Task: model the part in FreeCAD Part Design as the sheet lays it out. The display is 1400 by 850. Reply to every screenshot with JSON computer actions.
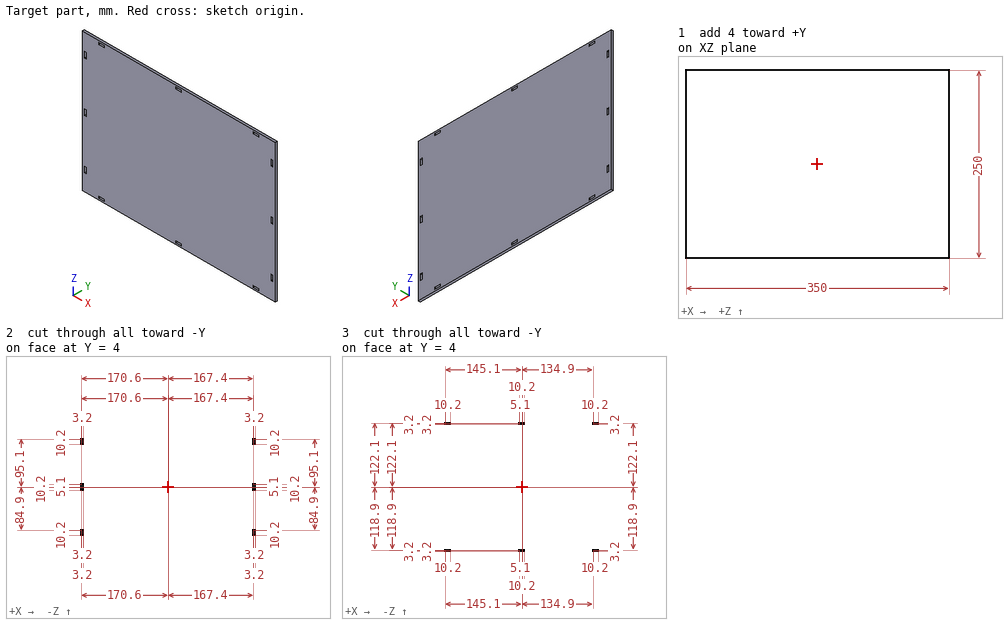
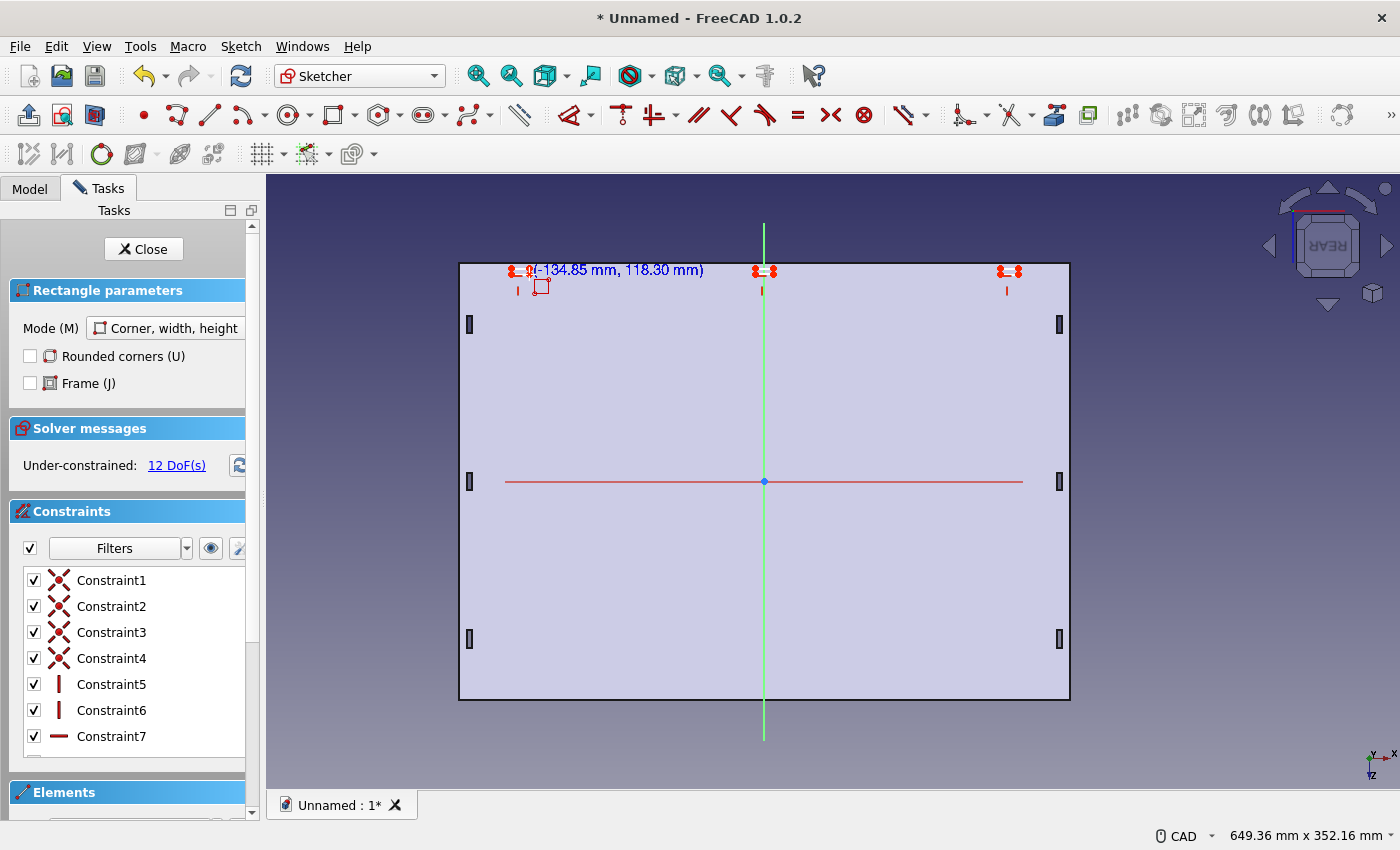
{"action": "scroll", "coordinate": [511, 689], "scroll_direction": "up", "scroll_amount": 6}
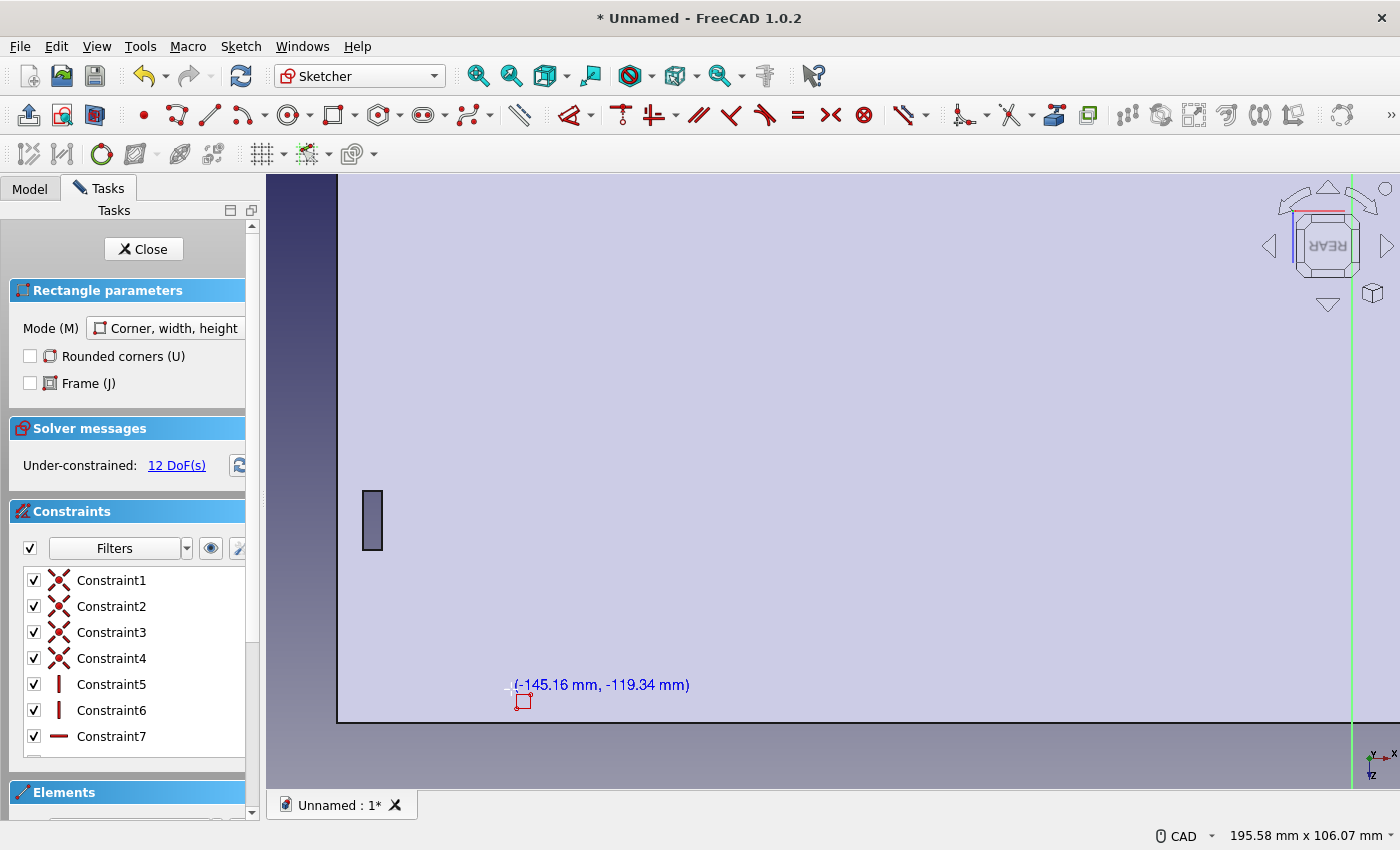
{"action": "scroll", "coordinate": [511, 690], "scroll_direction": "down", "scroll_amount": 6}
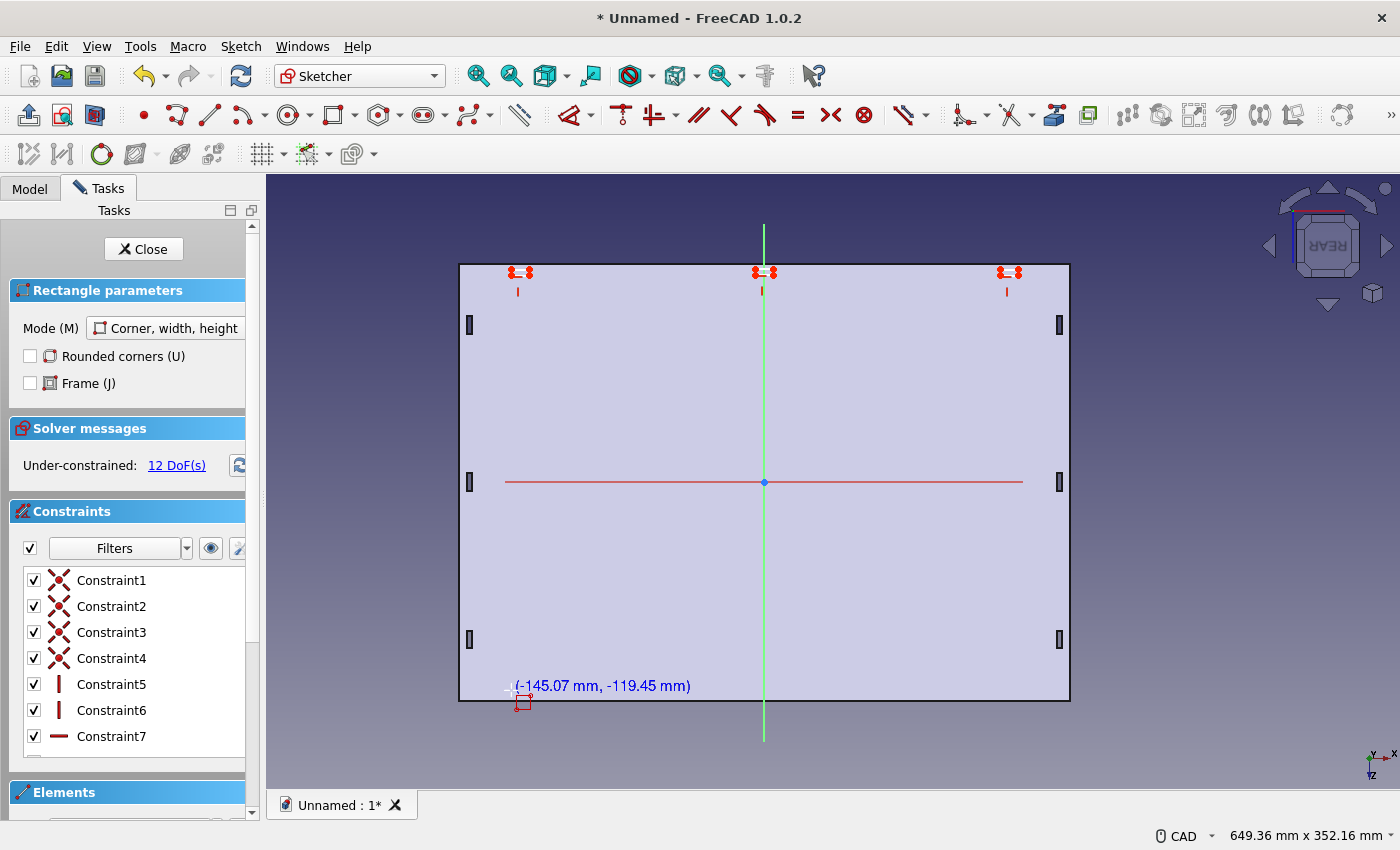
{"action": "left_click", "coordinate": [511, 690]}
{"action": "left_click", "coordinate": [529, 696]}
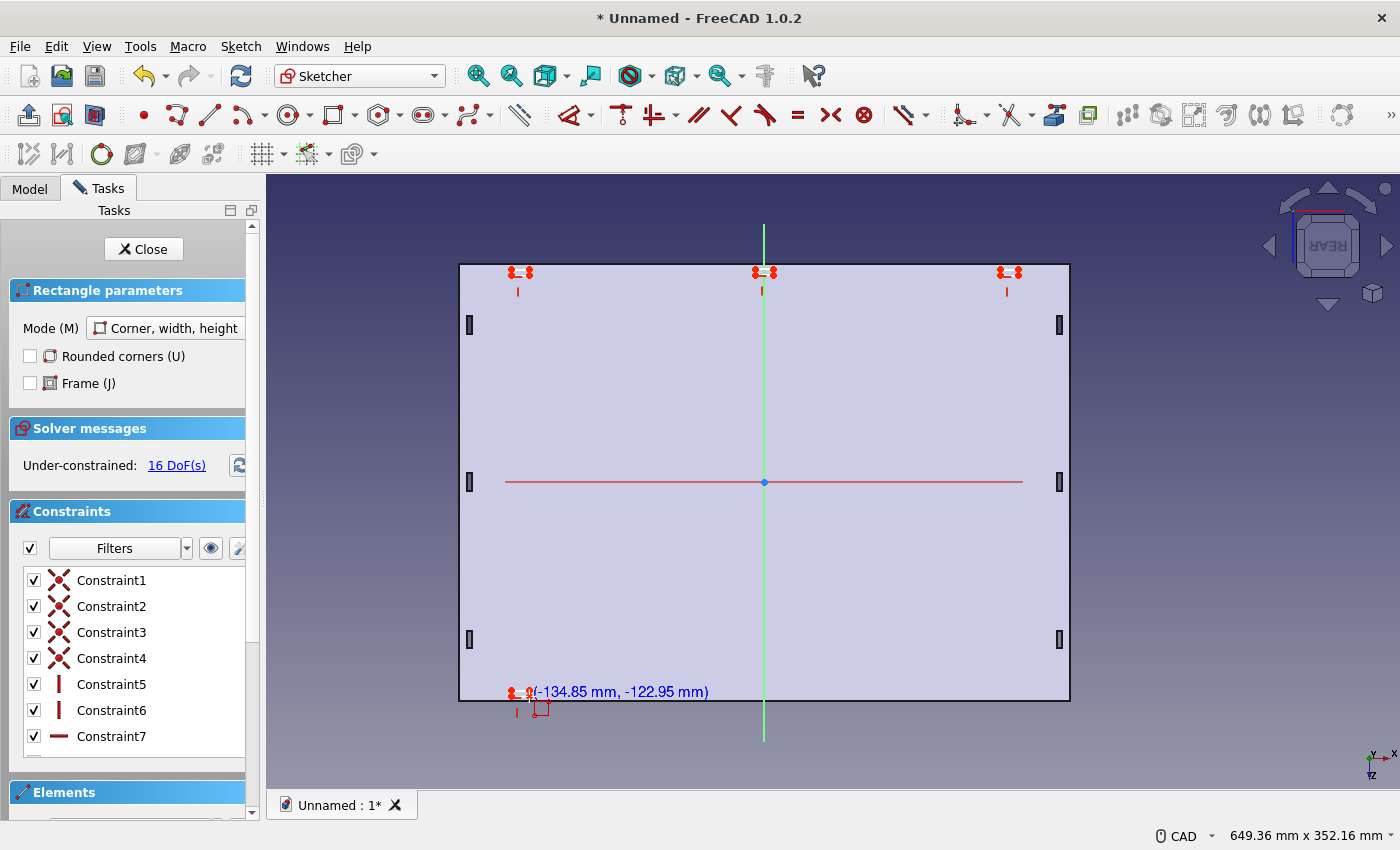
{"action": "scroll", "coordinate": [1000, 690], "scroll_direction": "up", "scroll_amount": 6}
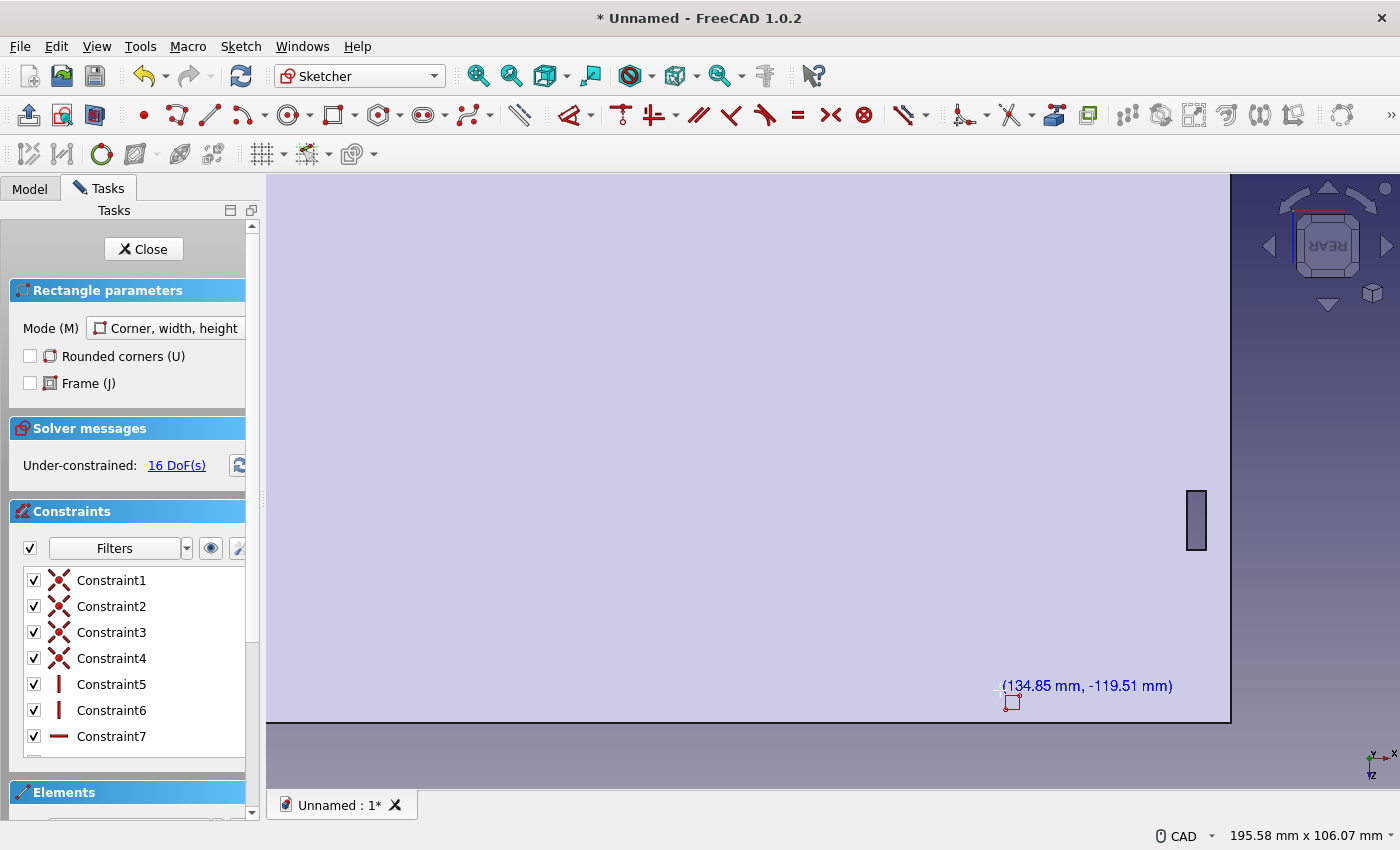
{"action": "scroll", "coordinate": [1001, 690], "scroll_direction": "down", "scroll_amount": 6}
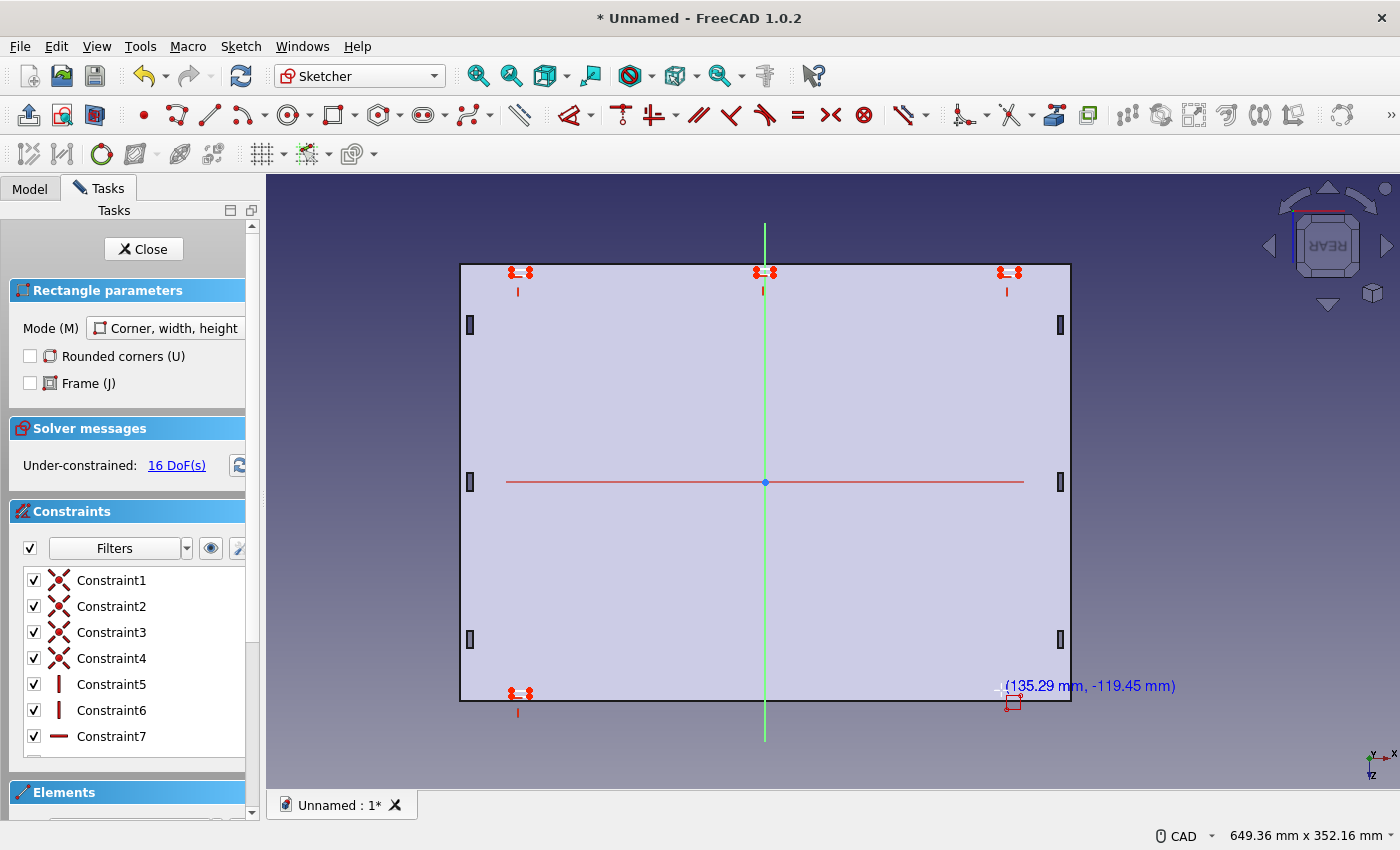
{"action": "left_click", "coordinate": [1001, 690]}
{"action": "left_click", "coordinate": [1019, 696]}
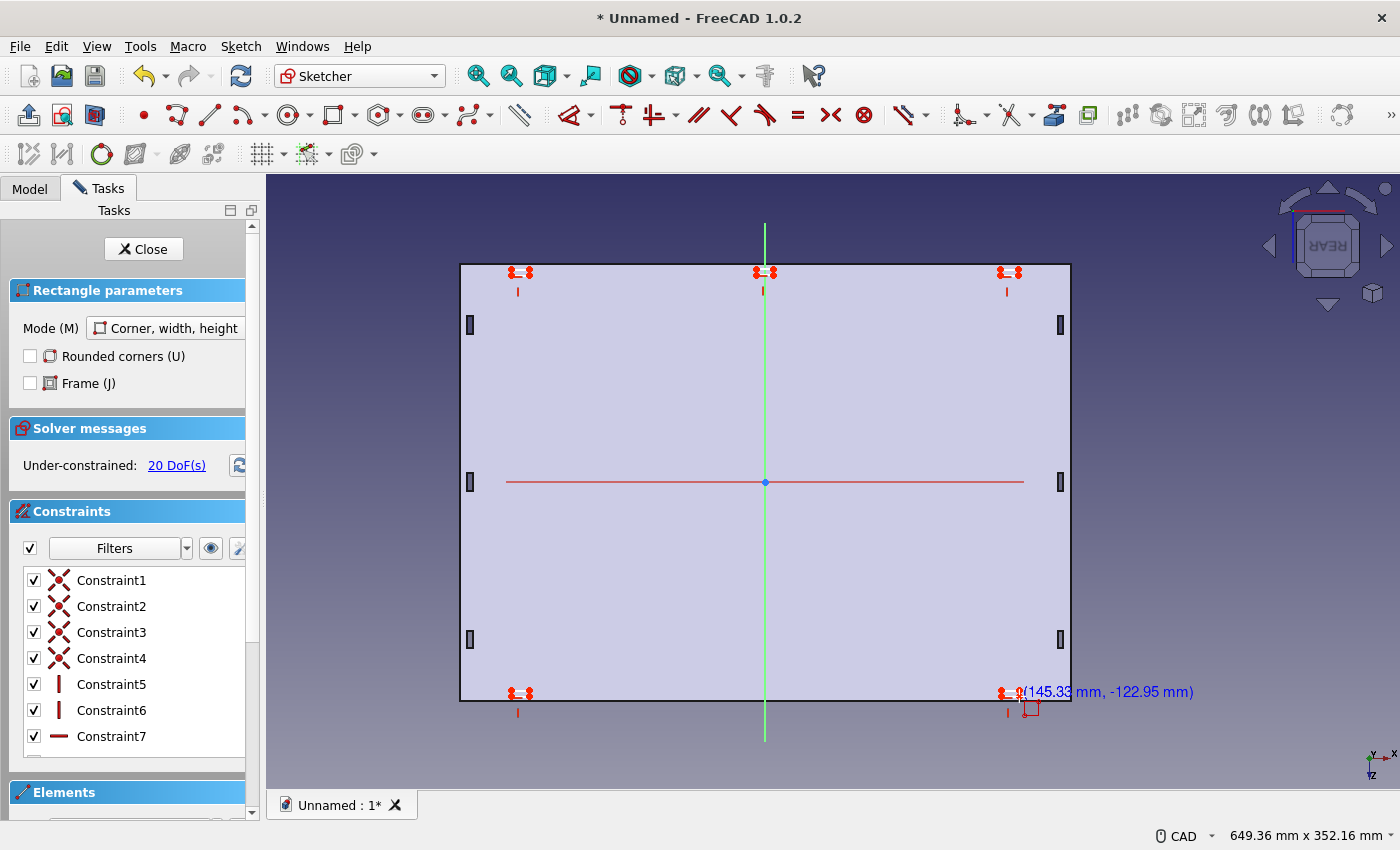
{"action": "scroll", "coordinate": [756, 690], "scroll_direction": "up", "scroll_amount": 6}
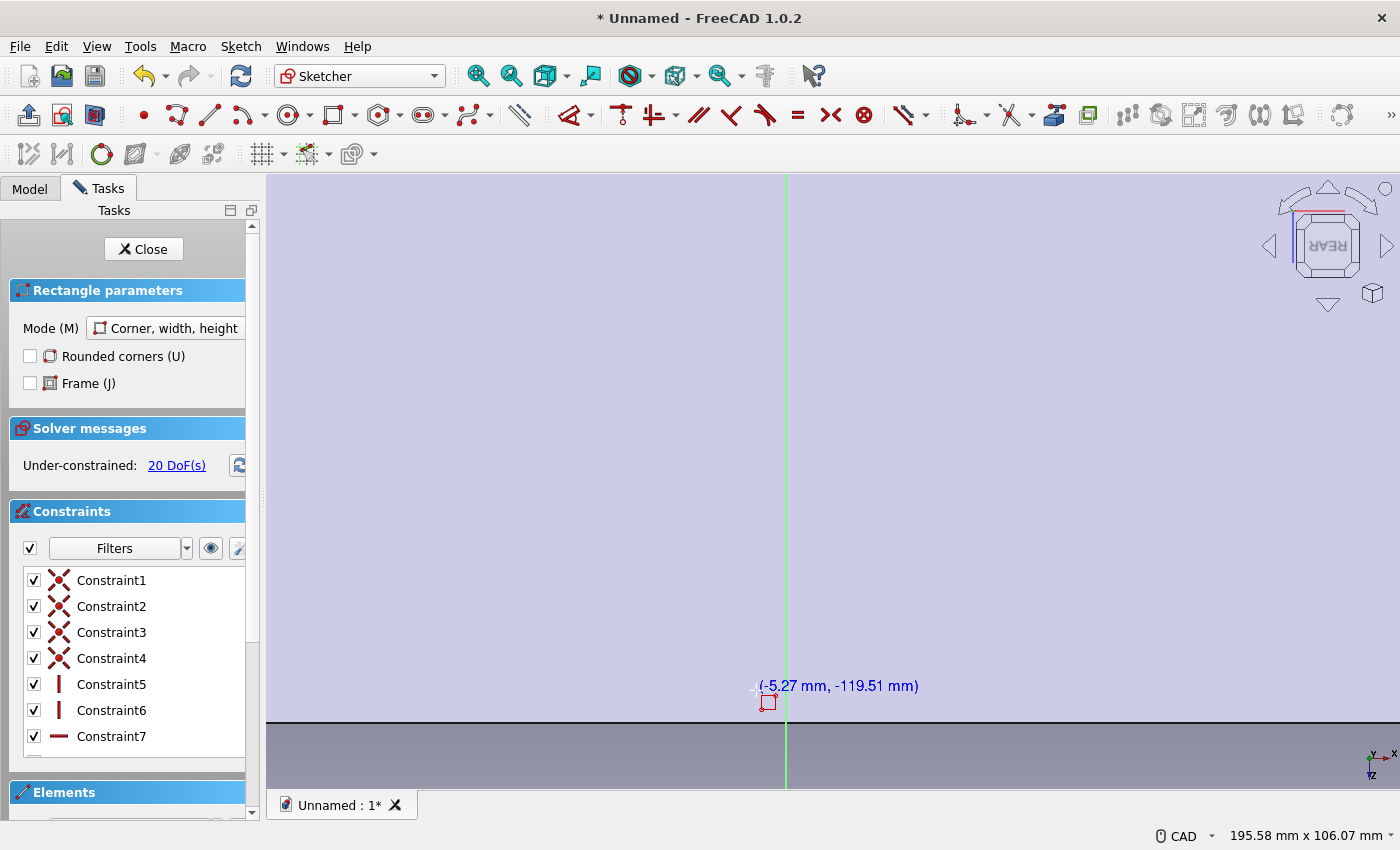
{"action": "left_click", "coordinate": [756, 688]}
{"action": "left_click", "coordinate": [815, 706]}
{"action": "key", "text": "Escape"}